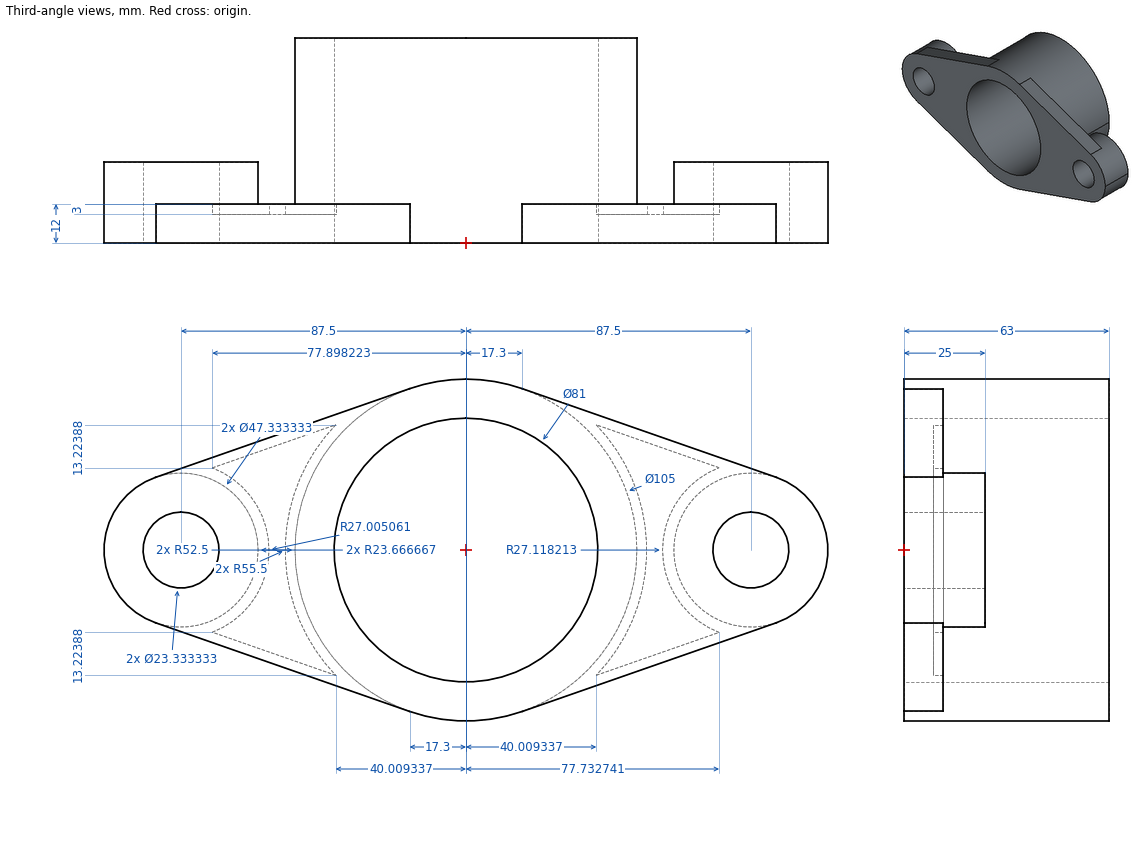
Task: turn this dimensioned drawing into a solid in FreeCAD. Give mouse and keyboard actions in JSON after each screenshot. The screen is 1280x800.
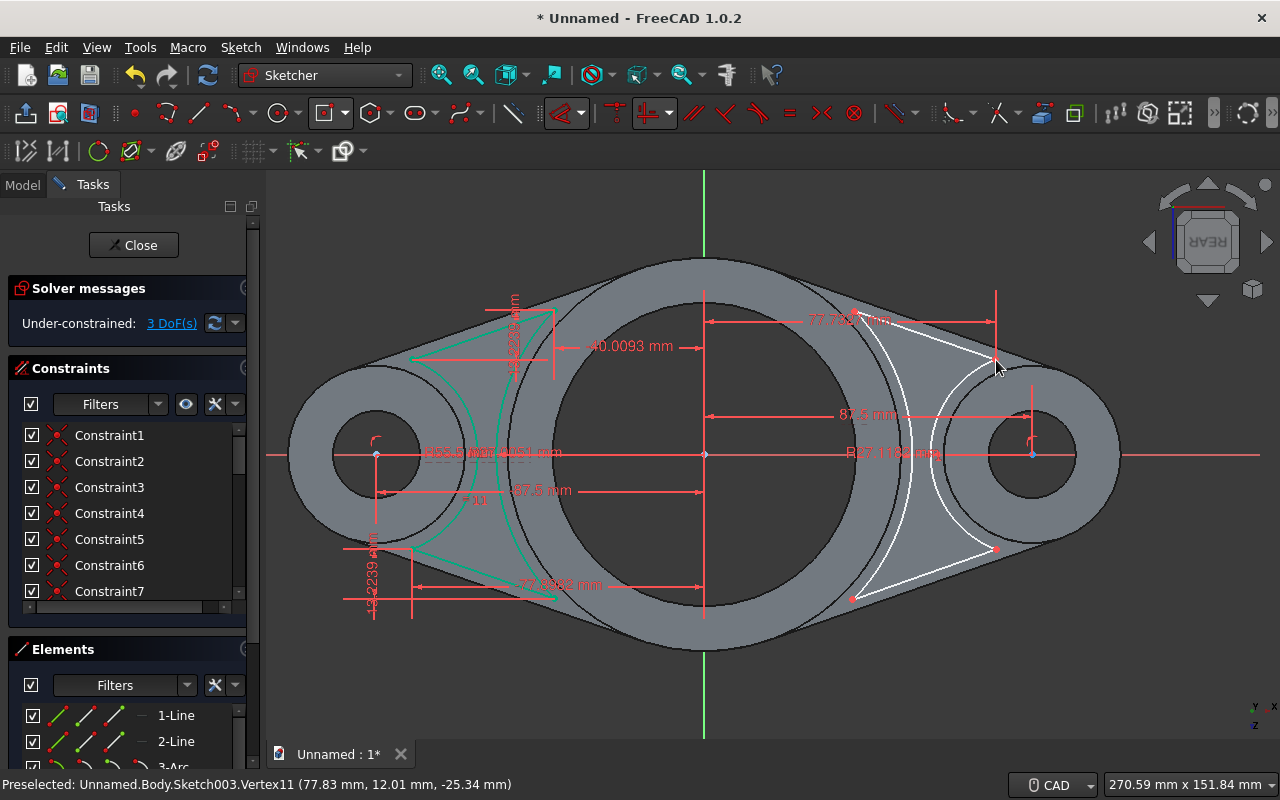
{"action": "left_click", "coordinate": [855, 311]}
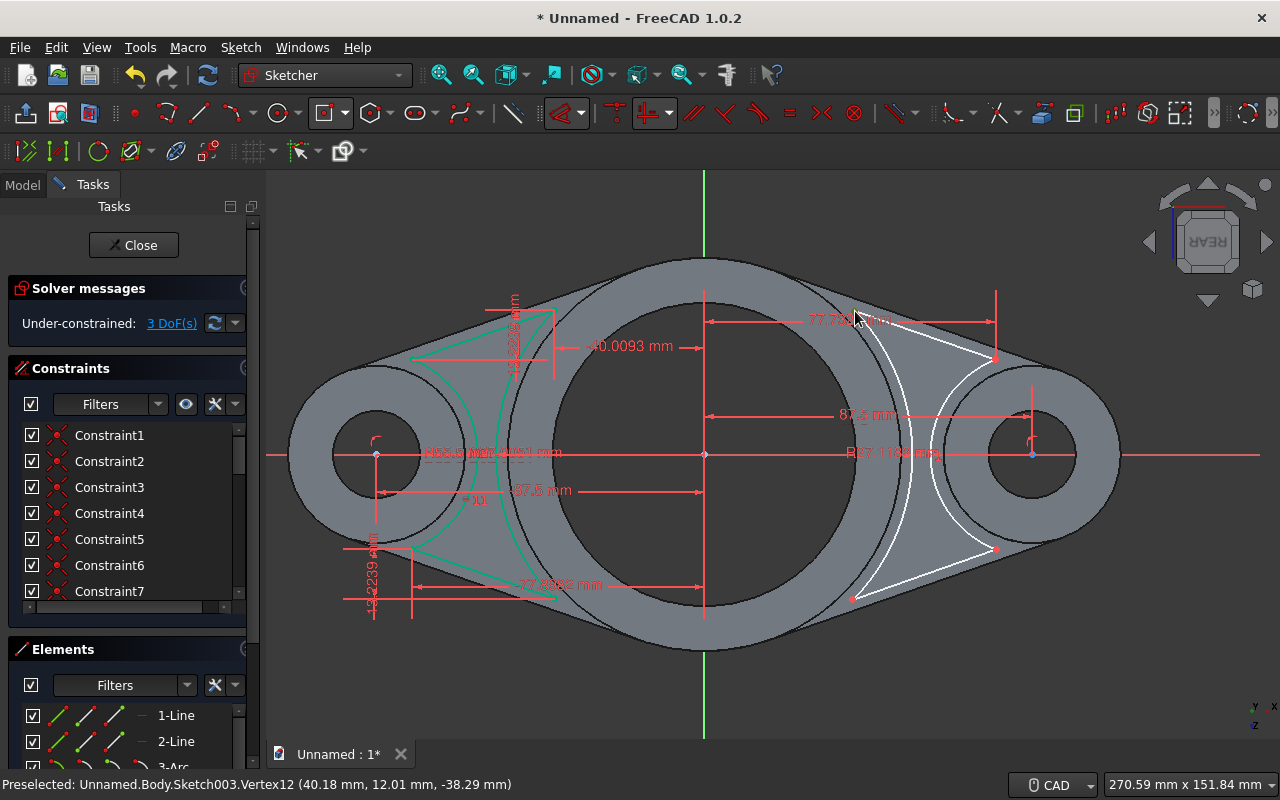
{"action": "key", "text": "l"}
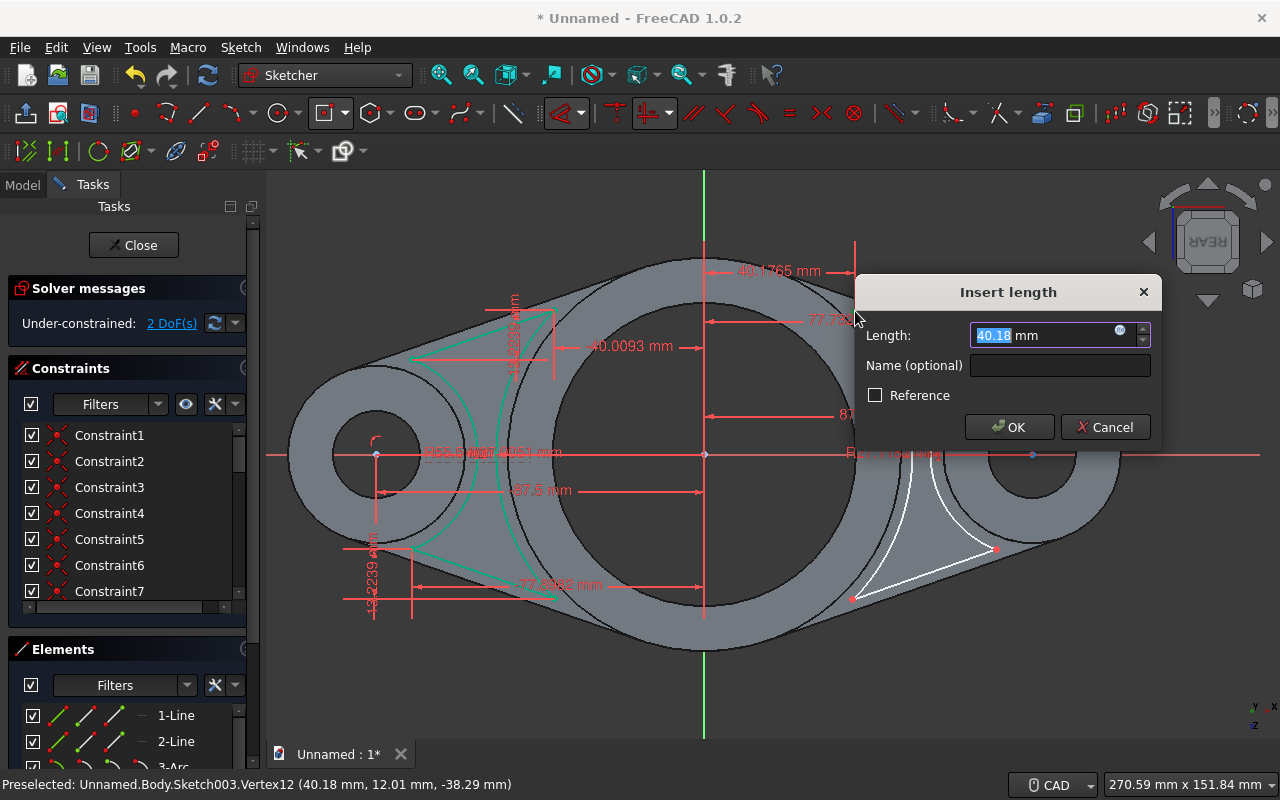
{"action": "type", "text": "40.009337"}
{"action": "key", "text": "Return"}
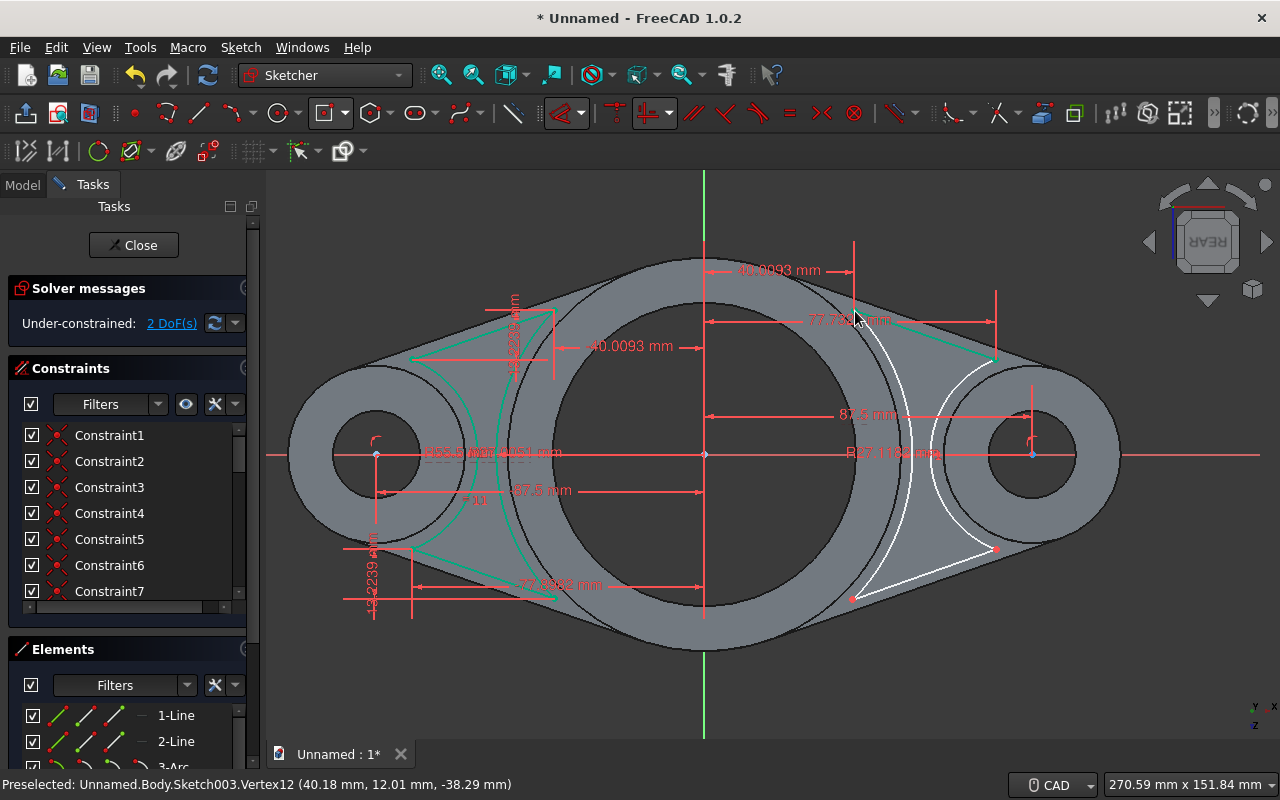
{"action": "left_click", "coordinate": [853, 600]}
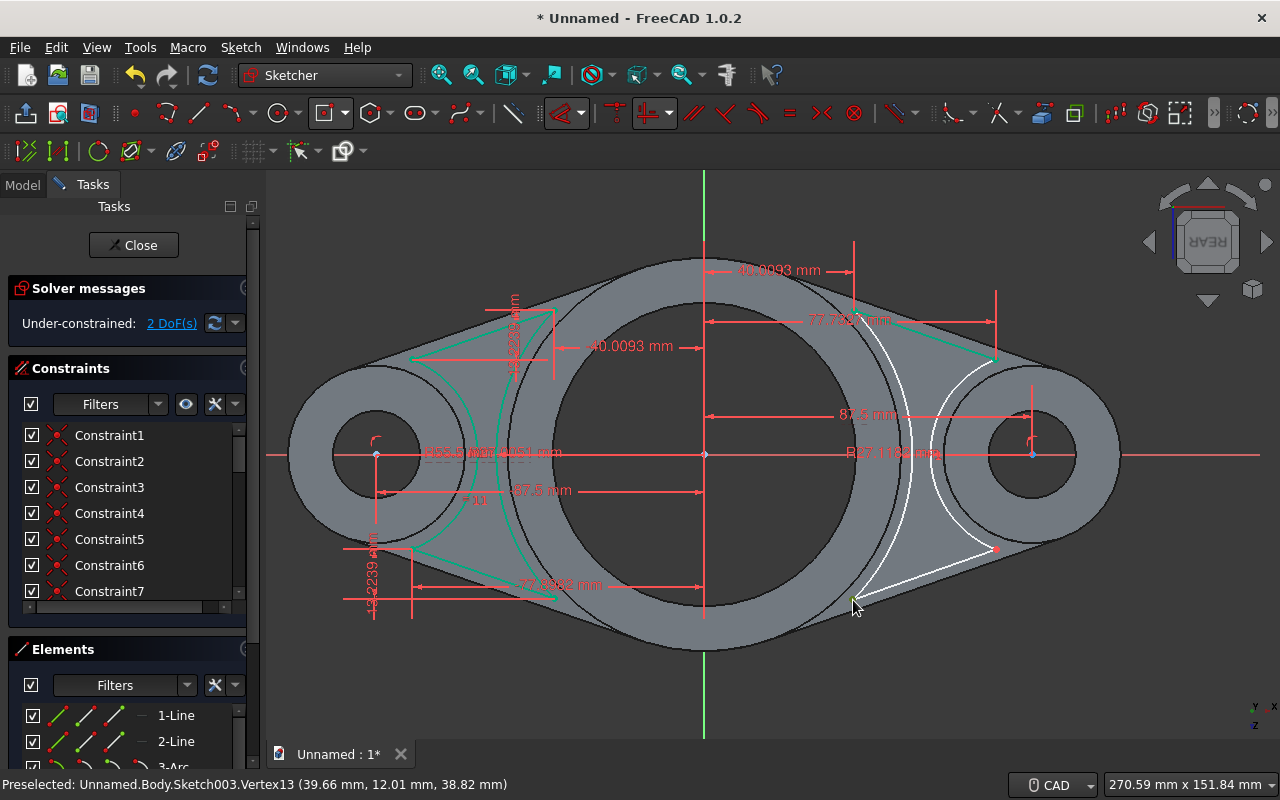
{"action": "key", "text": "l"}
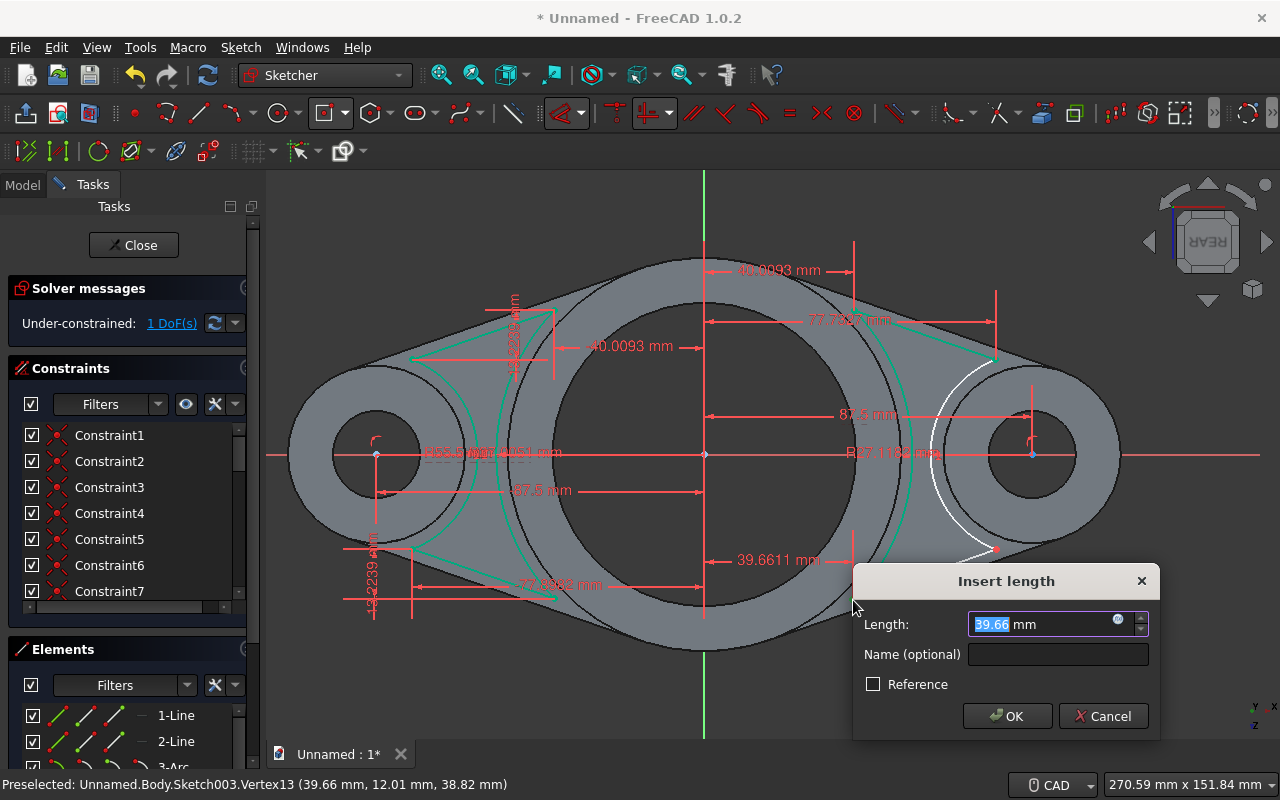
{"action": "type", "text": "40.009337"}
{"action": "key", "text": "Return"}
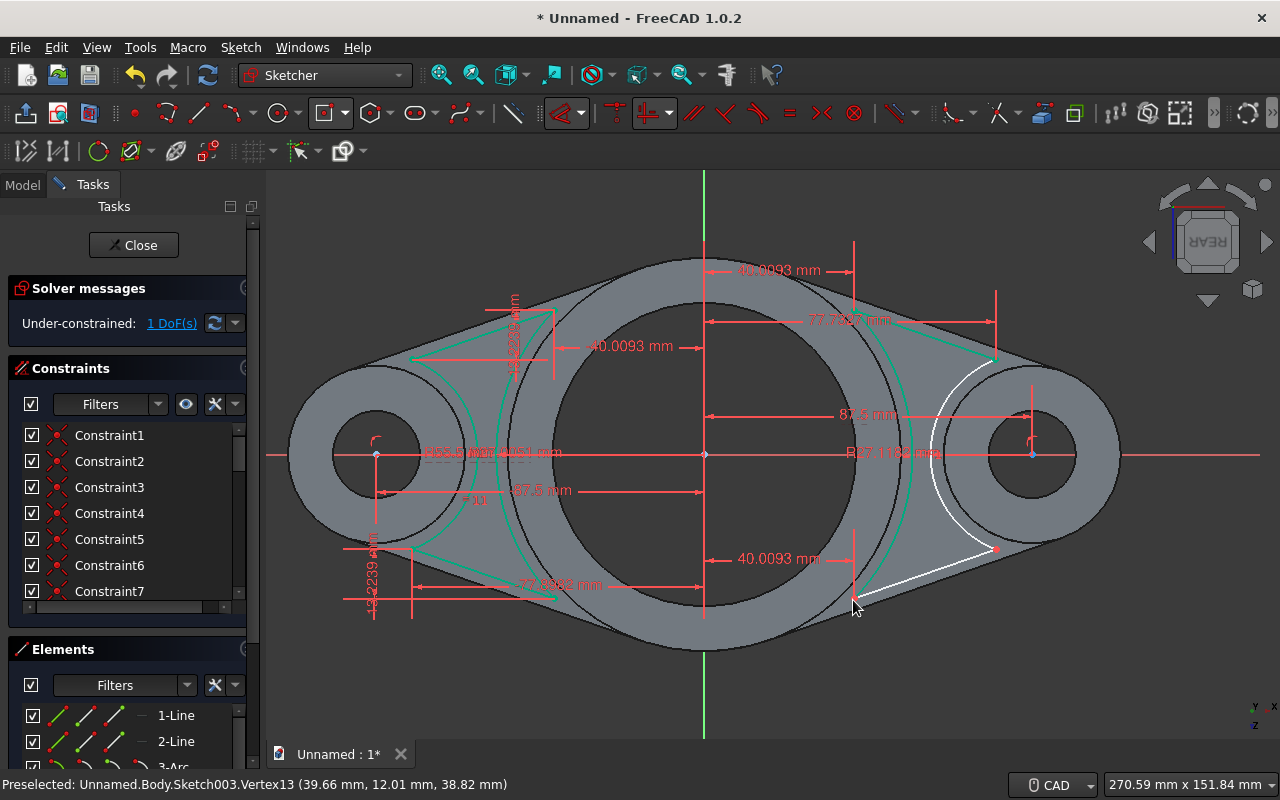
{"action": "left_click", "coordinate": [996, 549]}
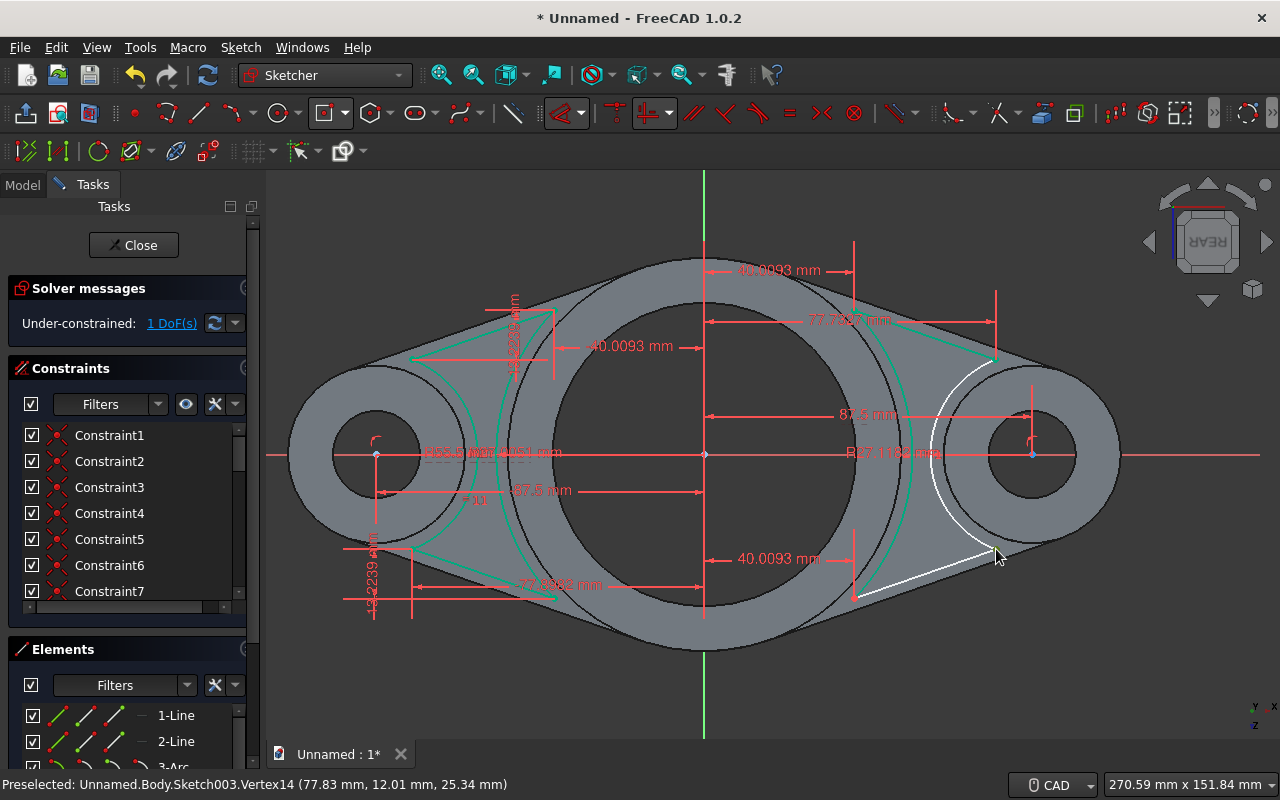
{"action": "key", "text": "l"}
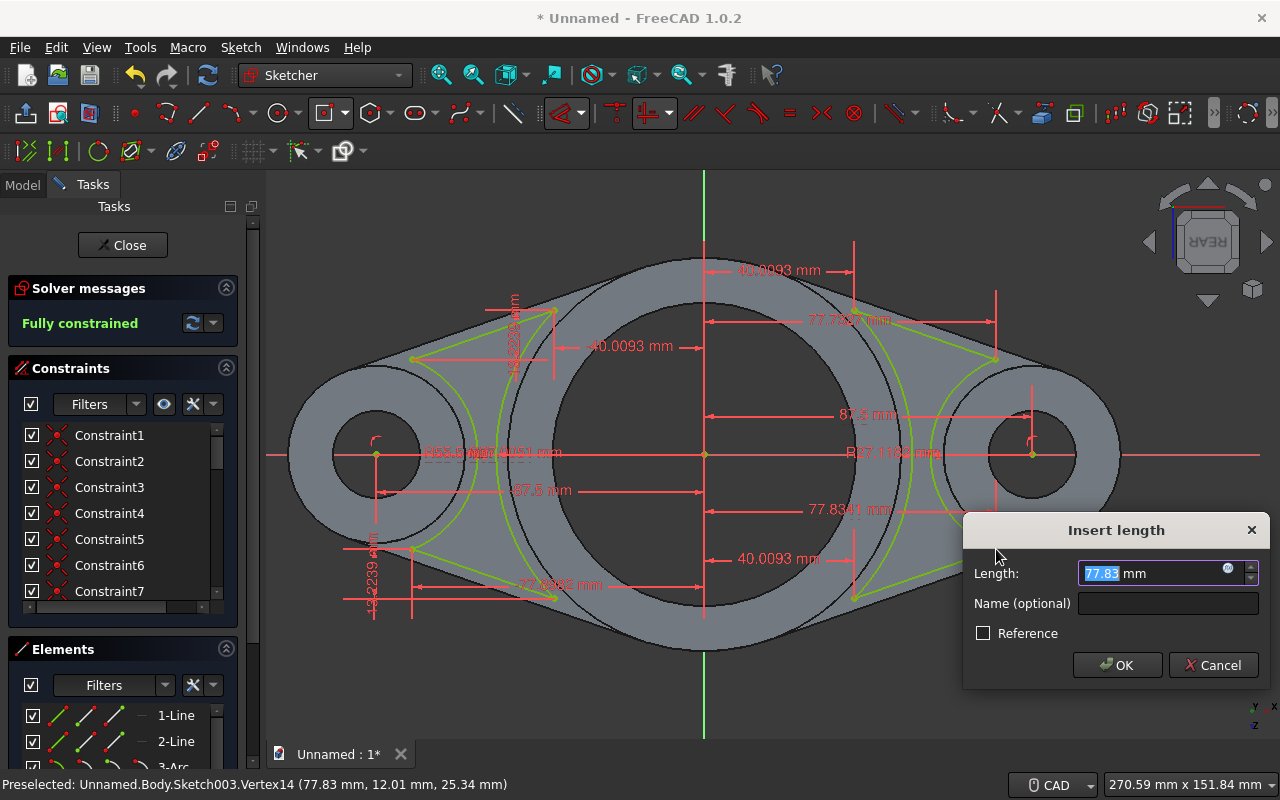
{"action": "type", "text": "77.732741"}
{"action": "key", "text": "Return"}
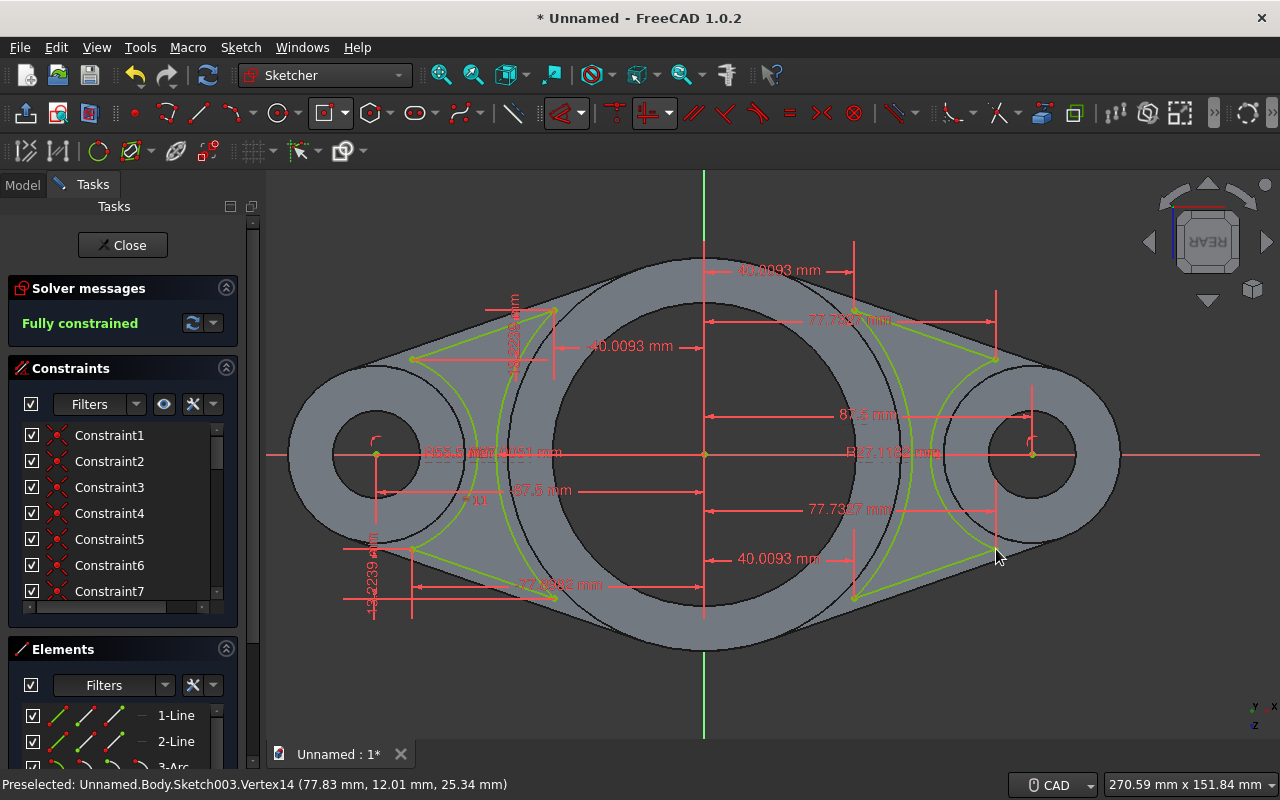
{"action": "left_click", "coordinate": [123, 245]}